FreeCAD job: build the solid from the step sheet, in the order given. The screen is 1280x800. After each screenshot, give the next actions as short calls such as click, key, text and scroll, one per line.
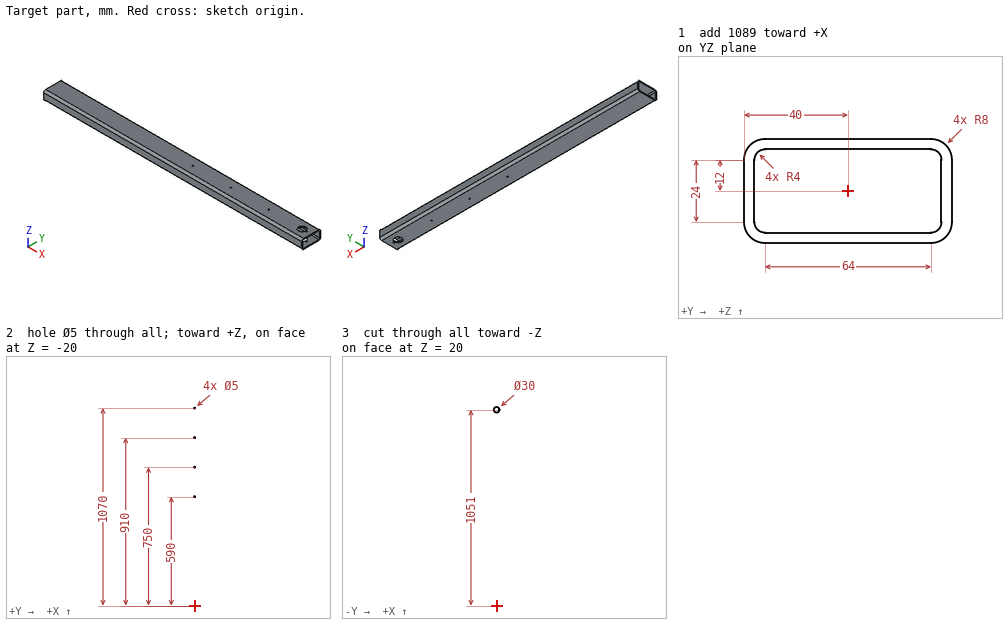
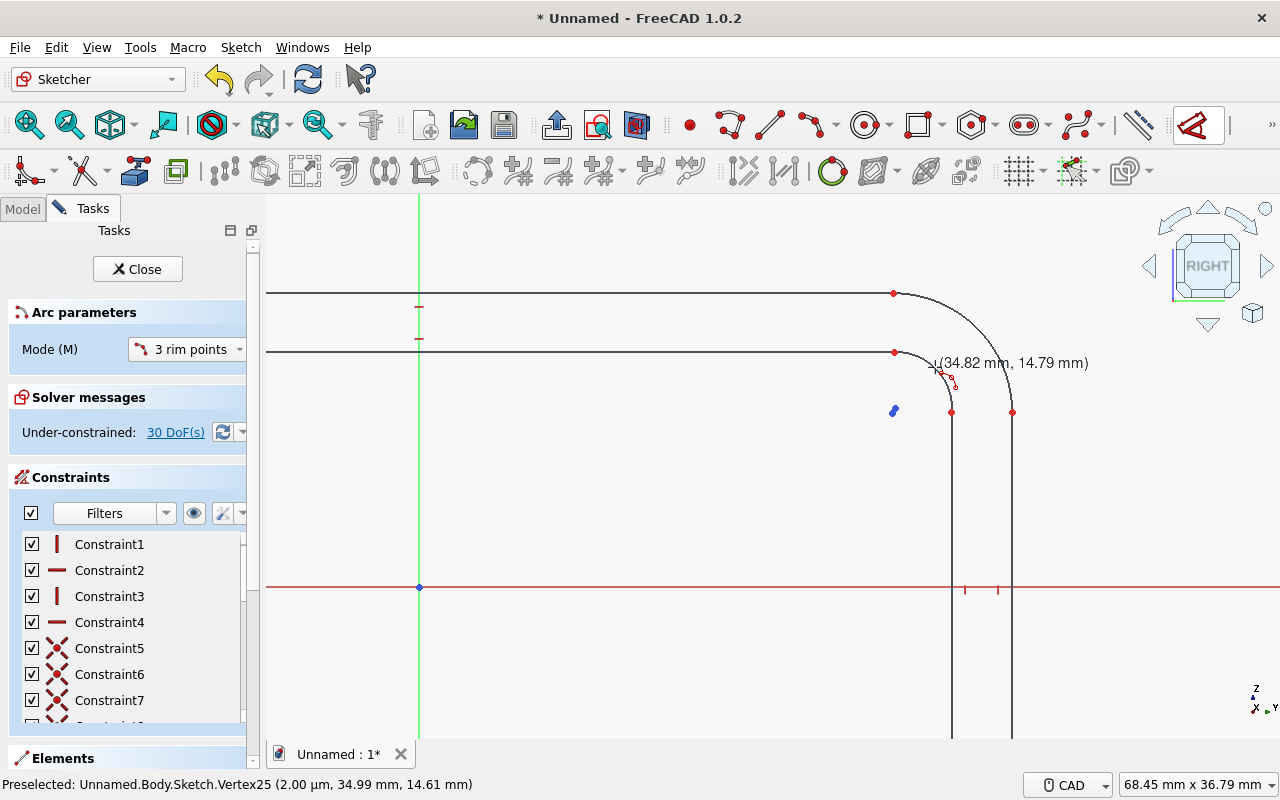
scroll(937, 368, down, 4)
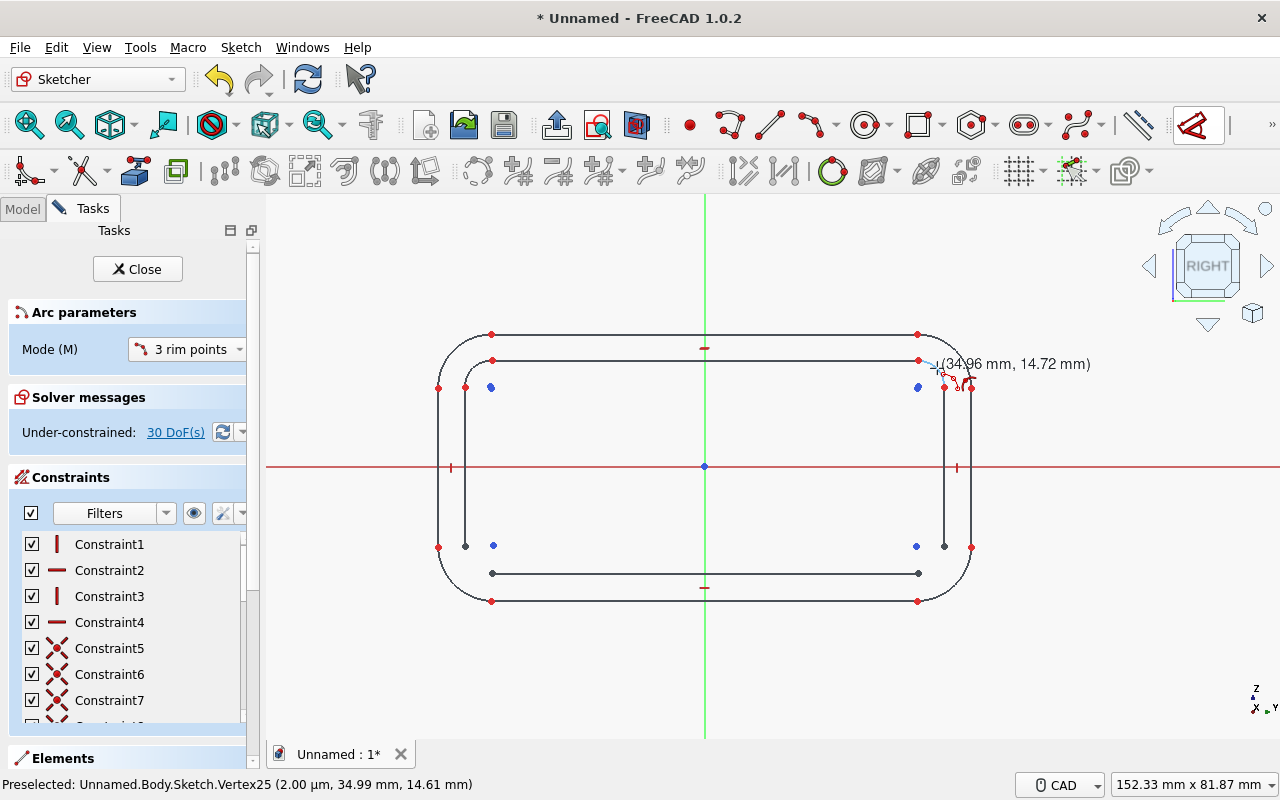
click(944, 547)
click(918, 574)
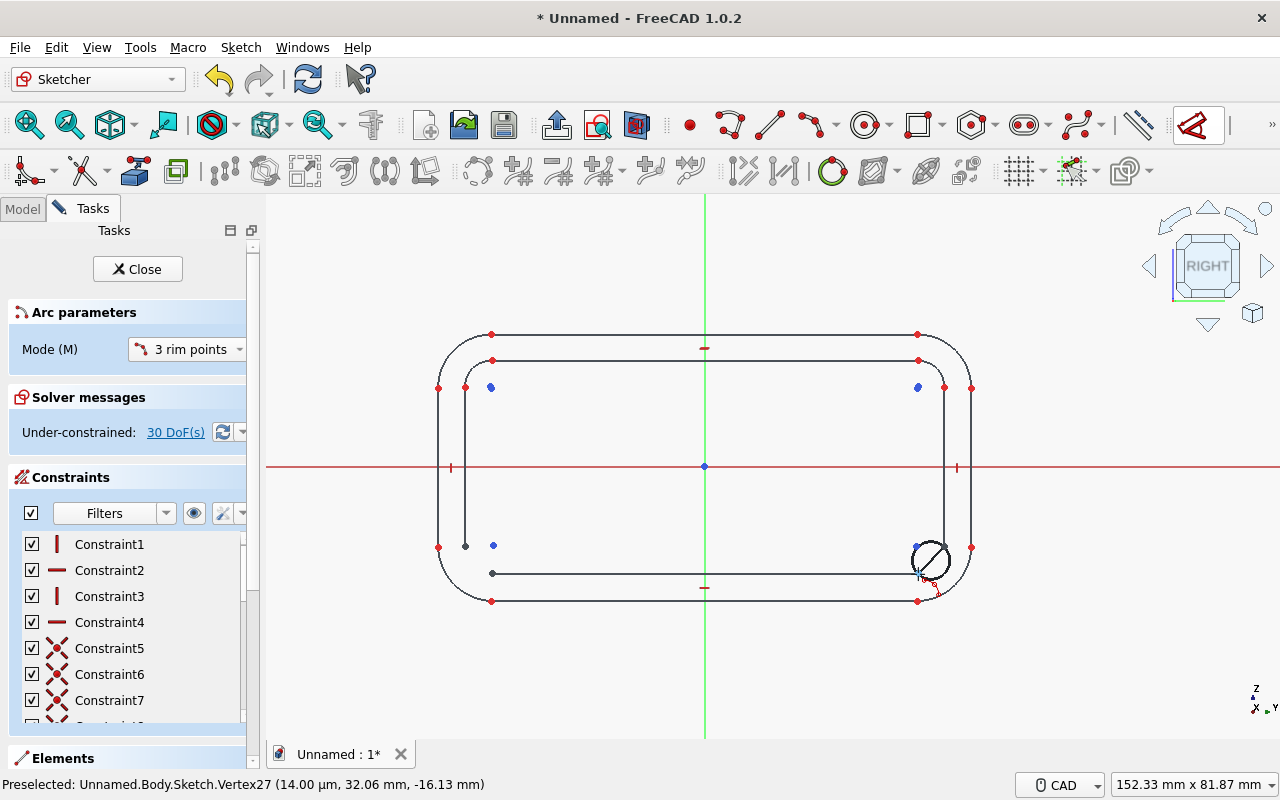
scroll(937, 565, up, 4)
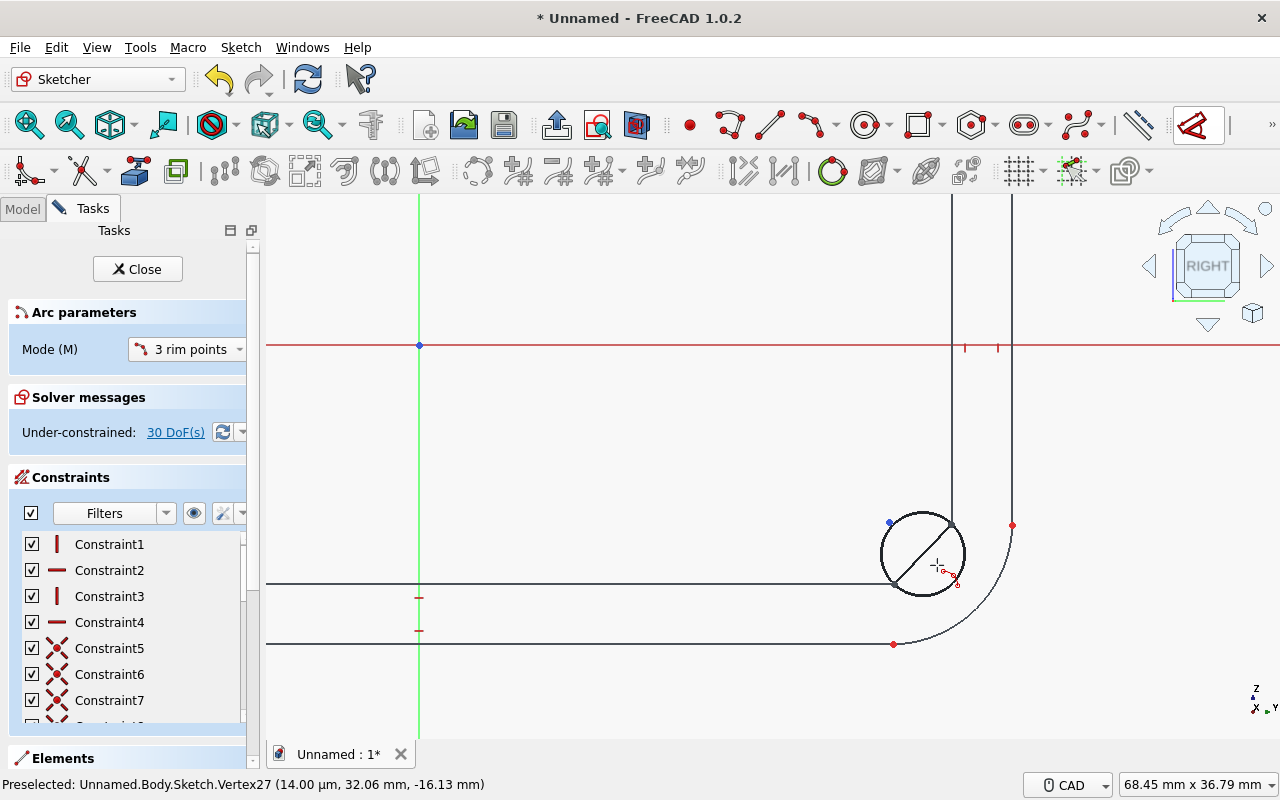
click(935, 565)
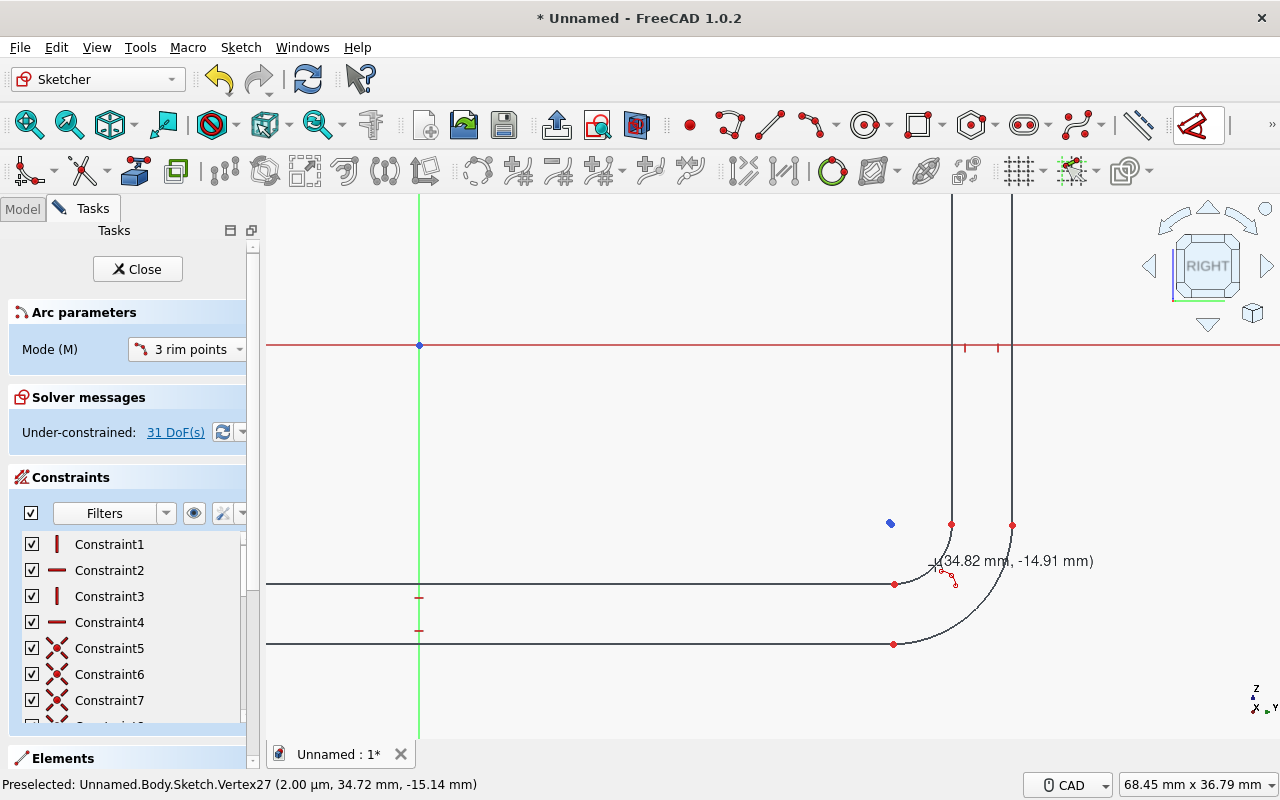
scroll(937, 566, down, 4)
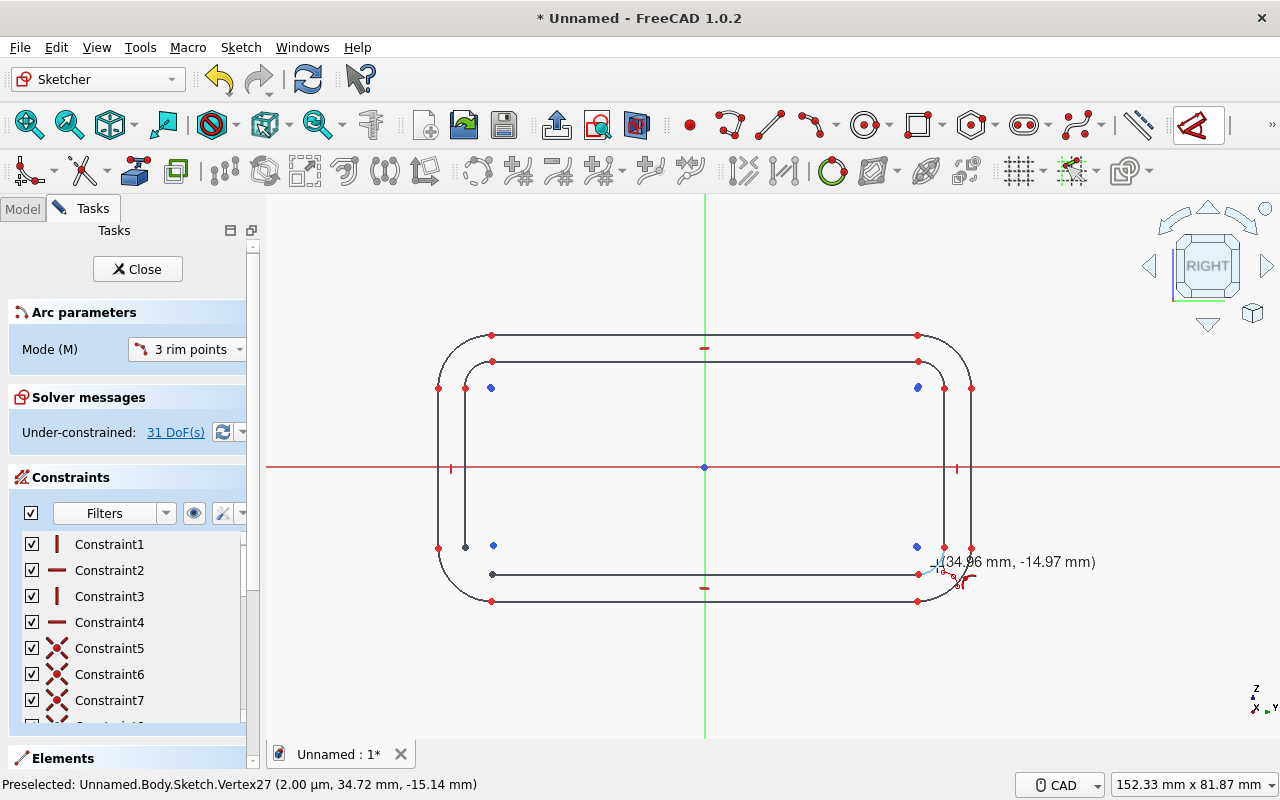
click(492, 575)
click(465, 548)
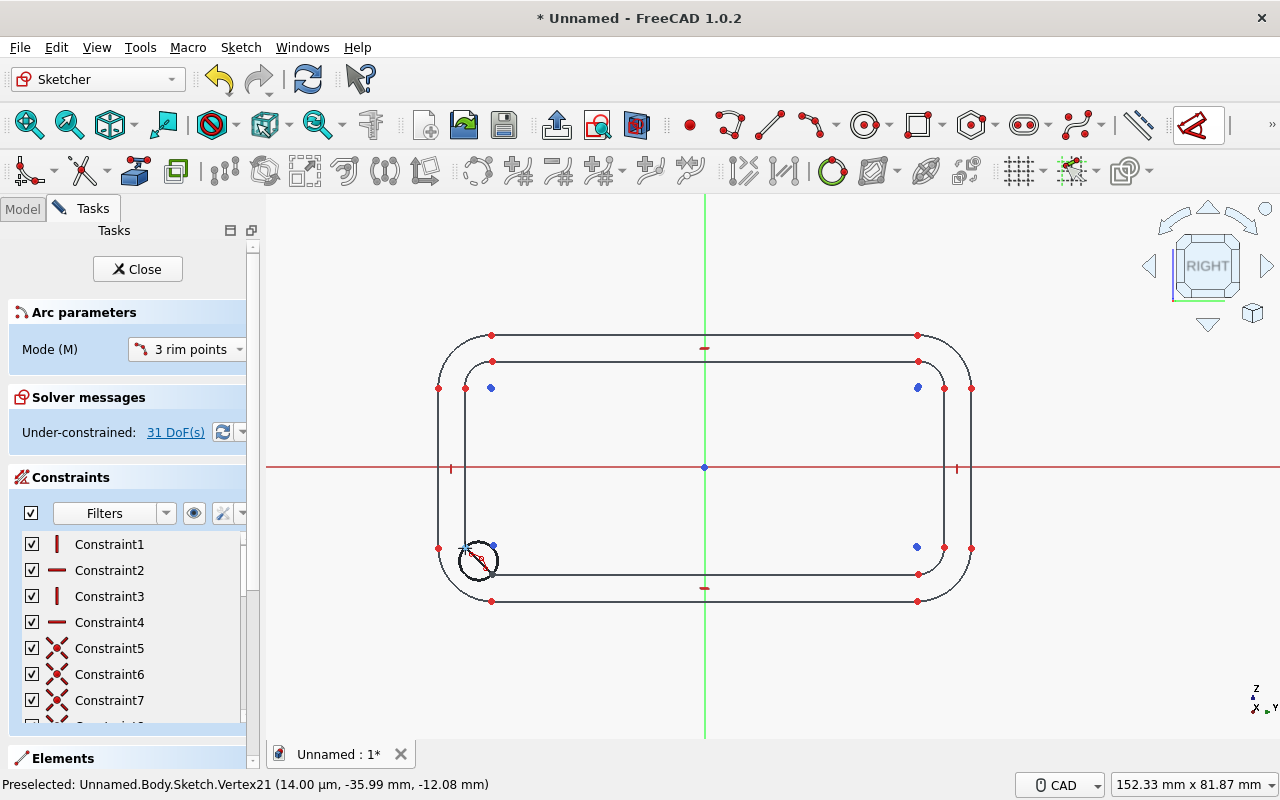
scroll(473, 566, up, 4)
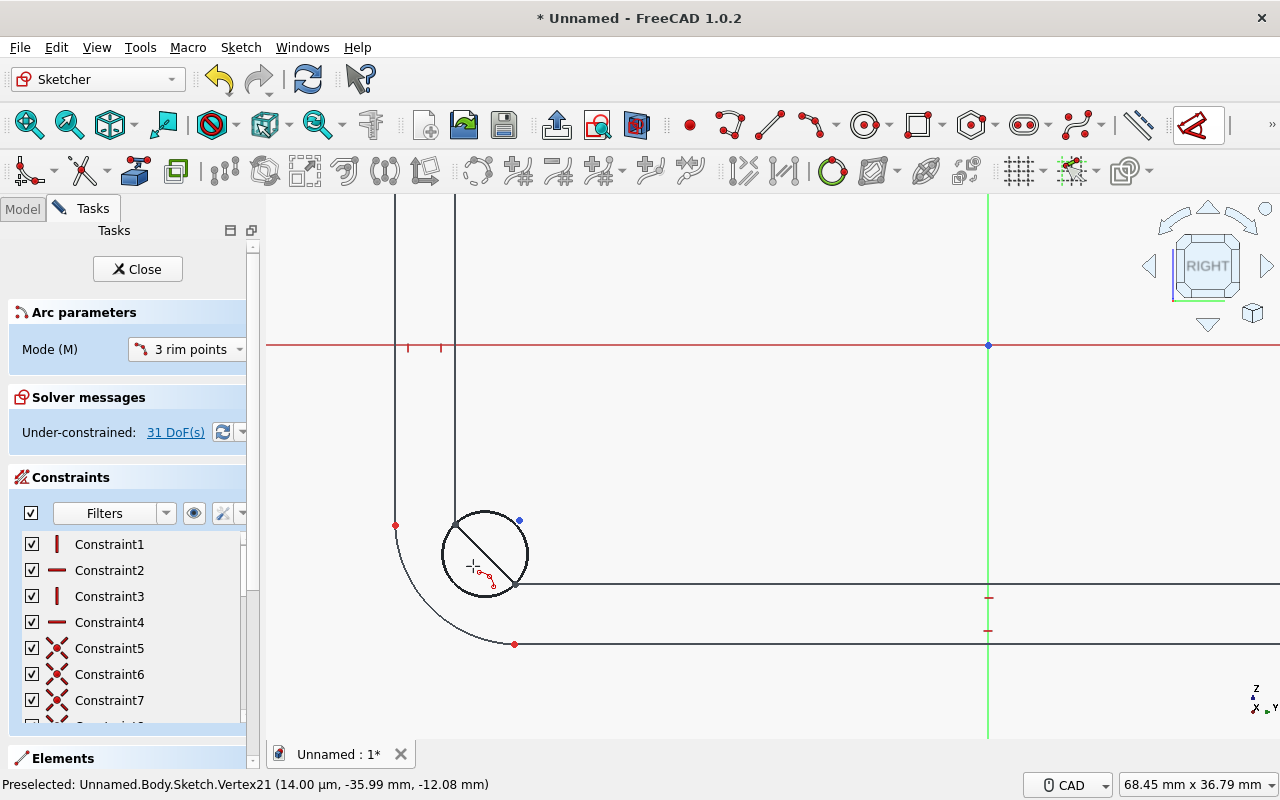
click(472, 565)
key(Escape)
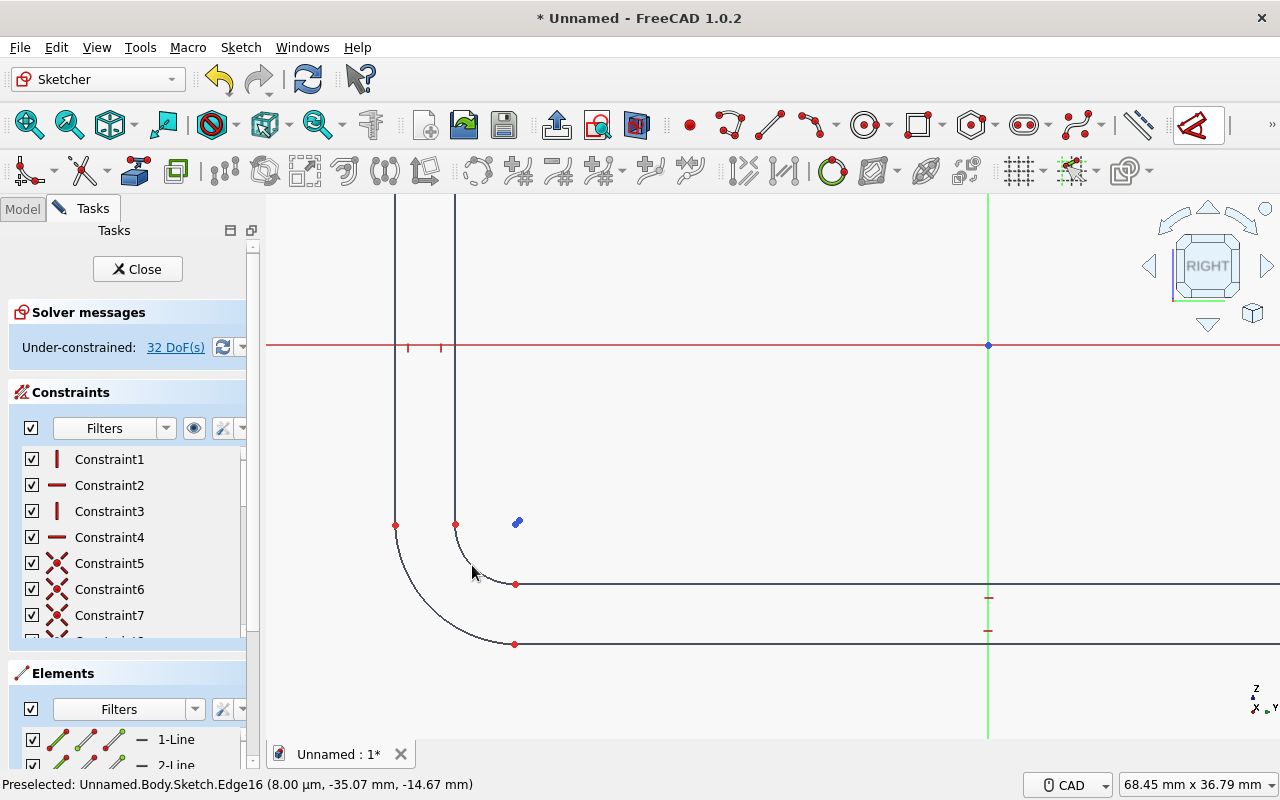
click(395, 277)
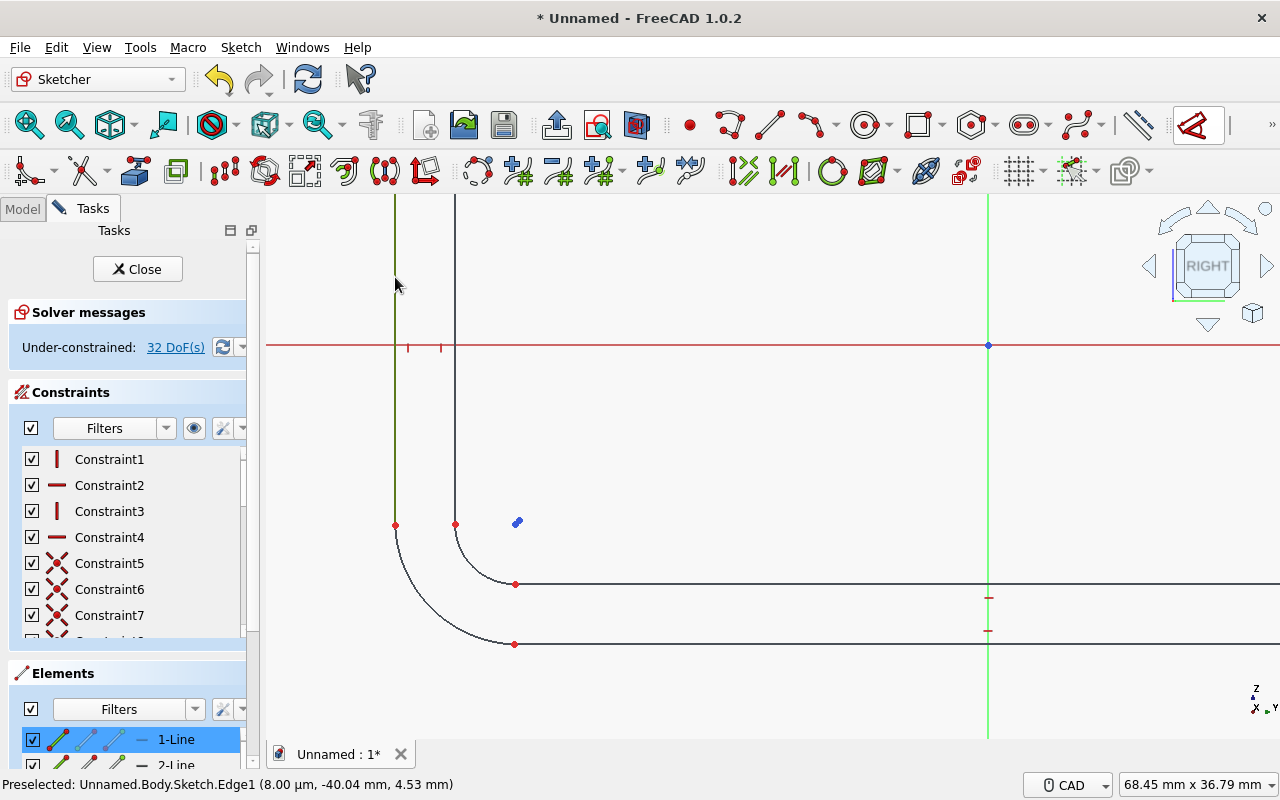
click(410, 578)